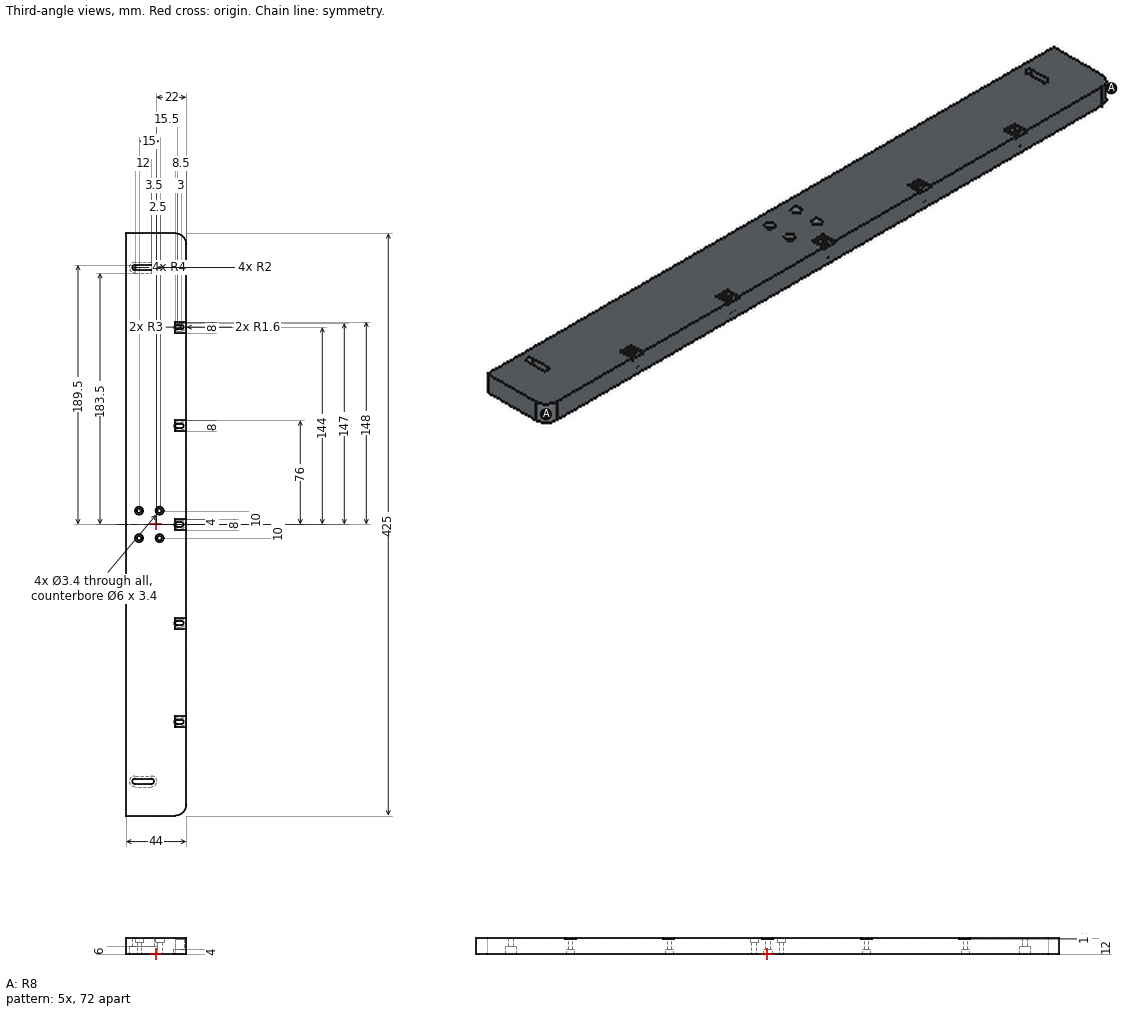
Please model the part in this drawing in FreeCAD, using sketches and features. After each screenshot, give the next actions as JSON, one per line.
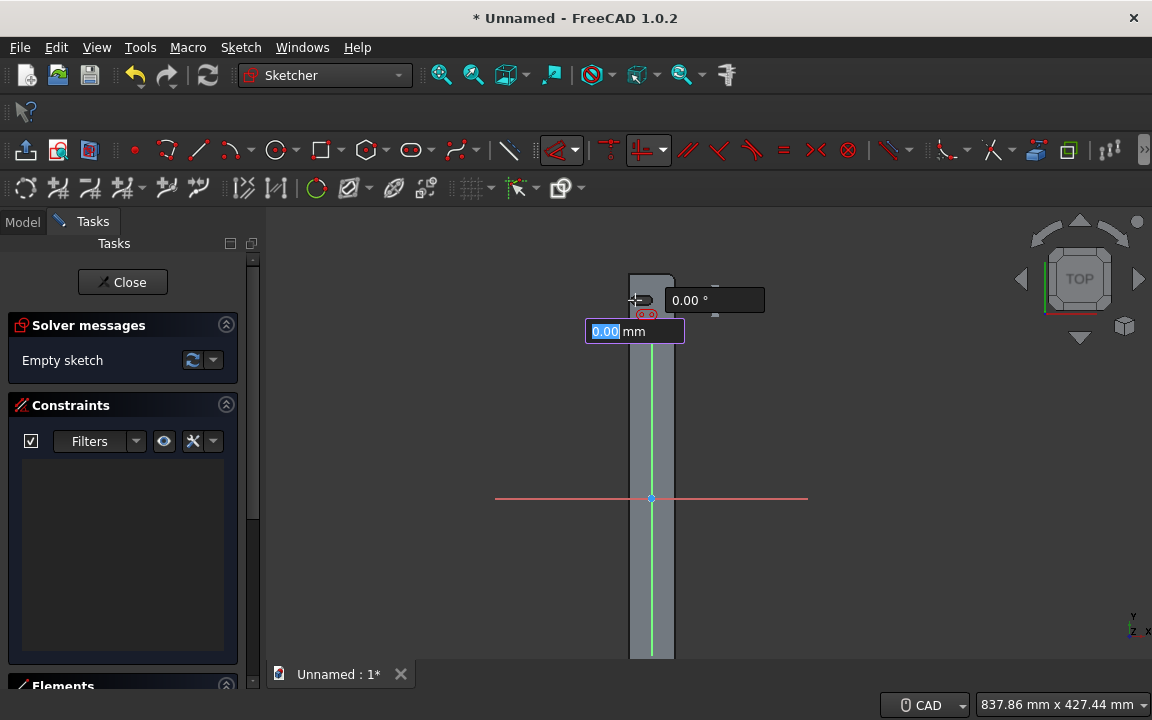
{"action": "scroll", "coordinate": [648, 300], "scroll_direction": "up", "scroll_amount": 8}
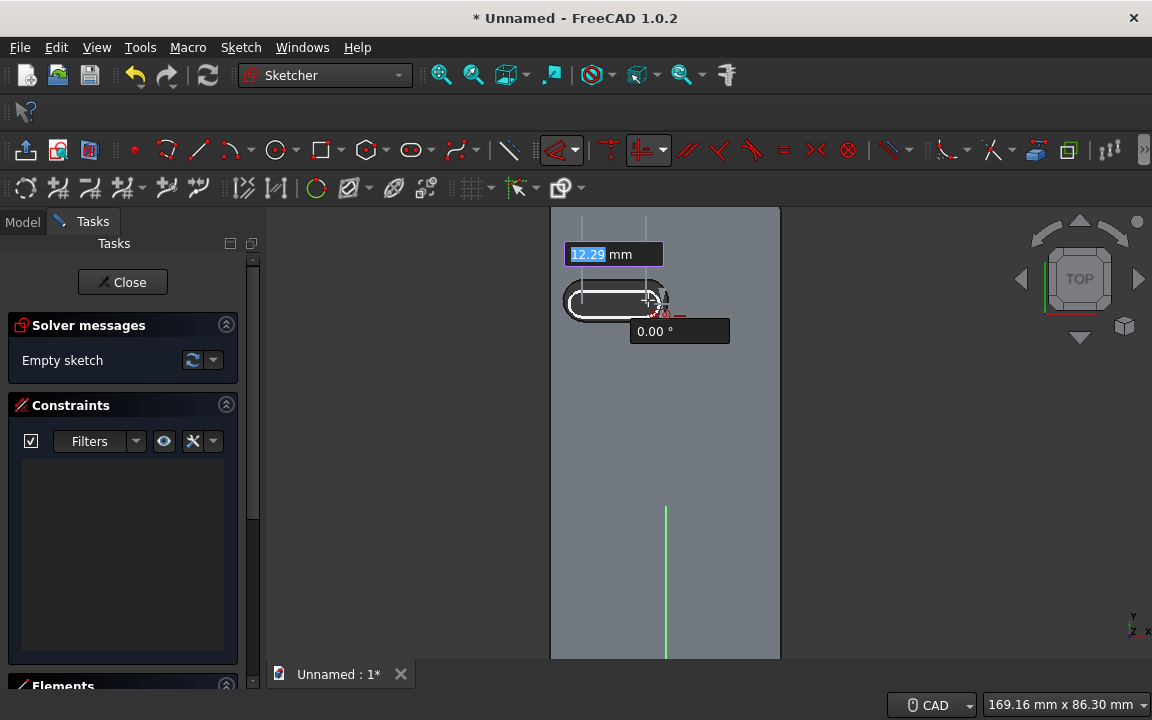
{"action": "left_click", "coordinate": [647, 299]}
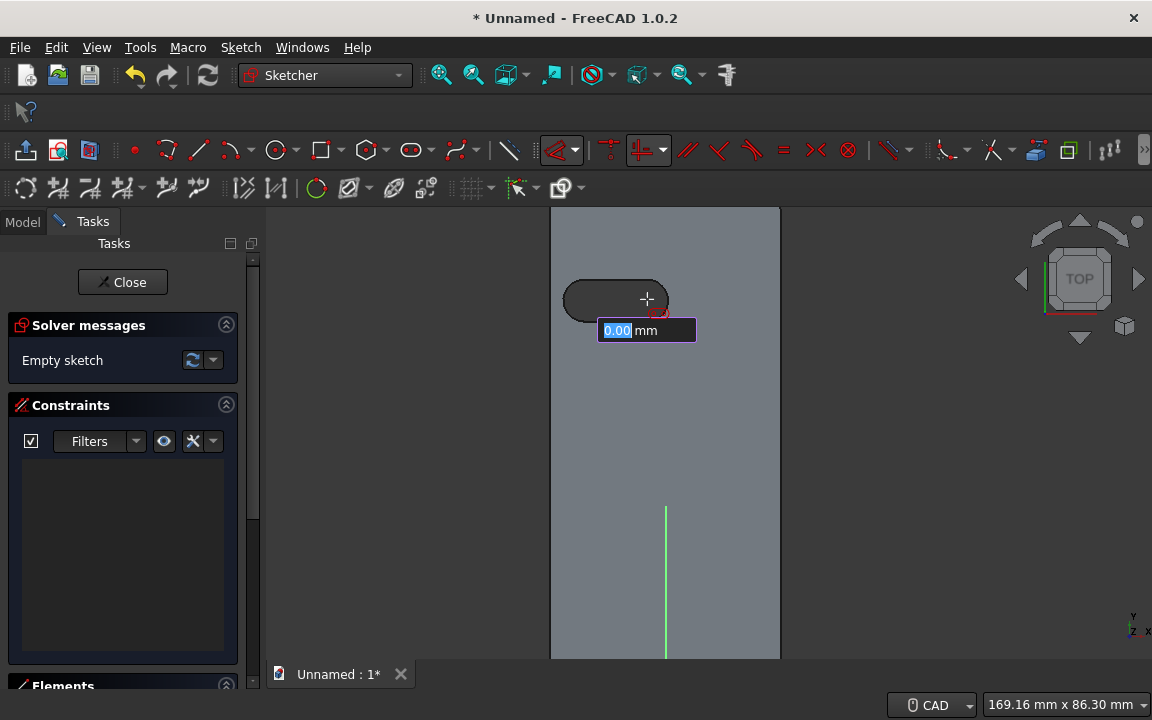
{"action": "scroll", "coordinate": [616, 290], "scroll_direction": "up", "scroll_amount": 3}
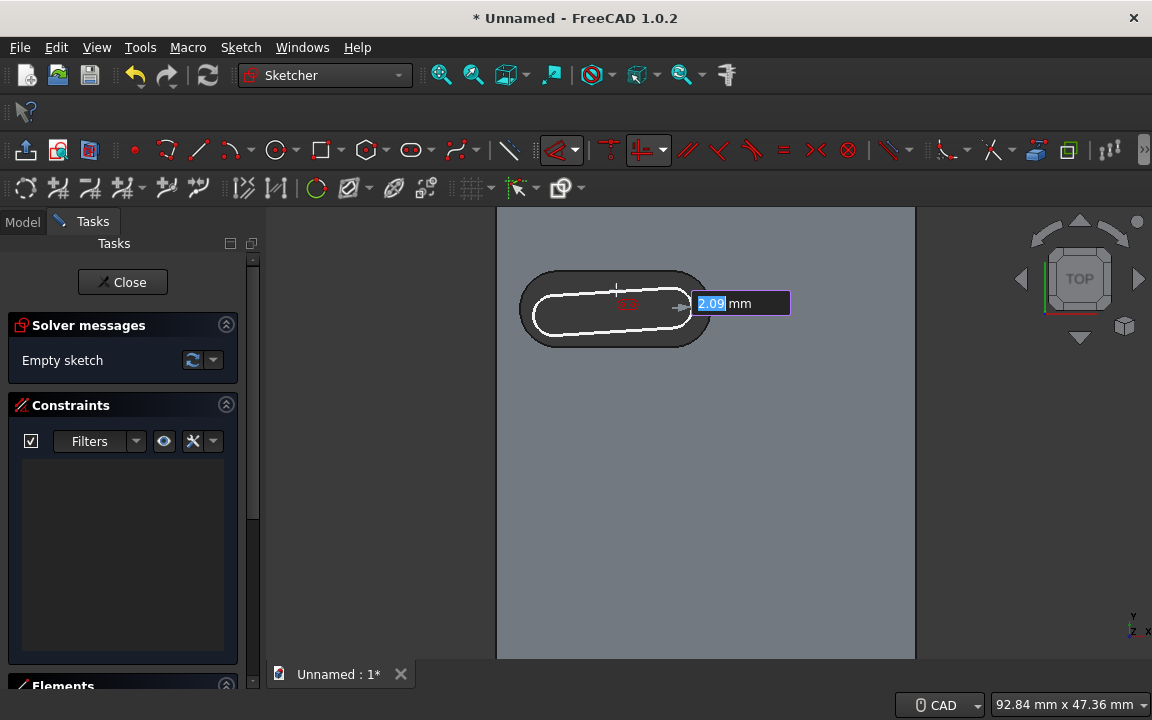
{"action": "left_click", "coordinate": [615, 290]}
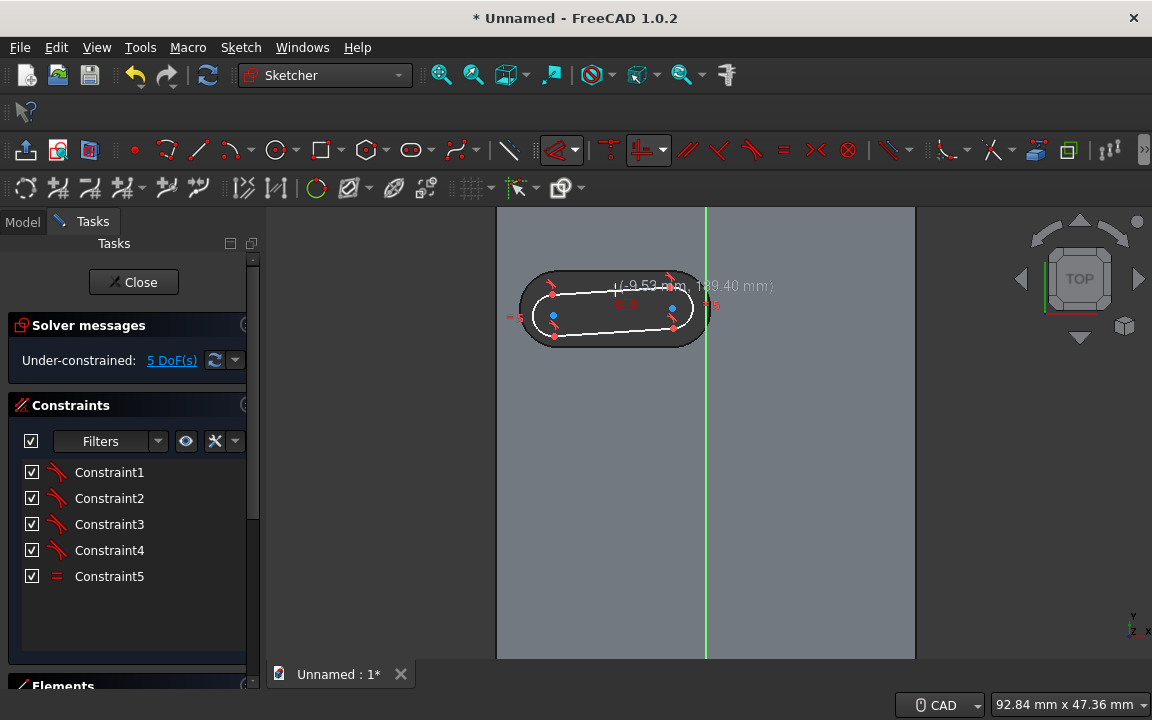
{"action": "scroll", "coordinate": [642, 299], "scroll_direction": "down", "scroll_amount": 13}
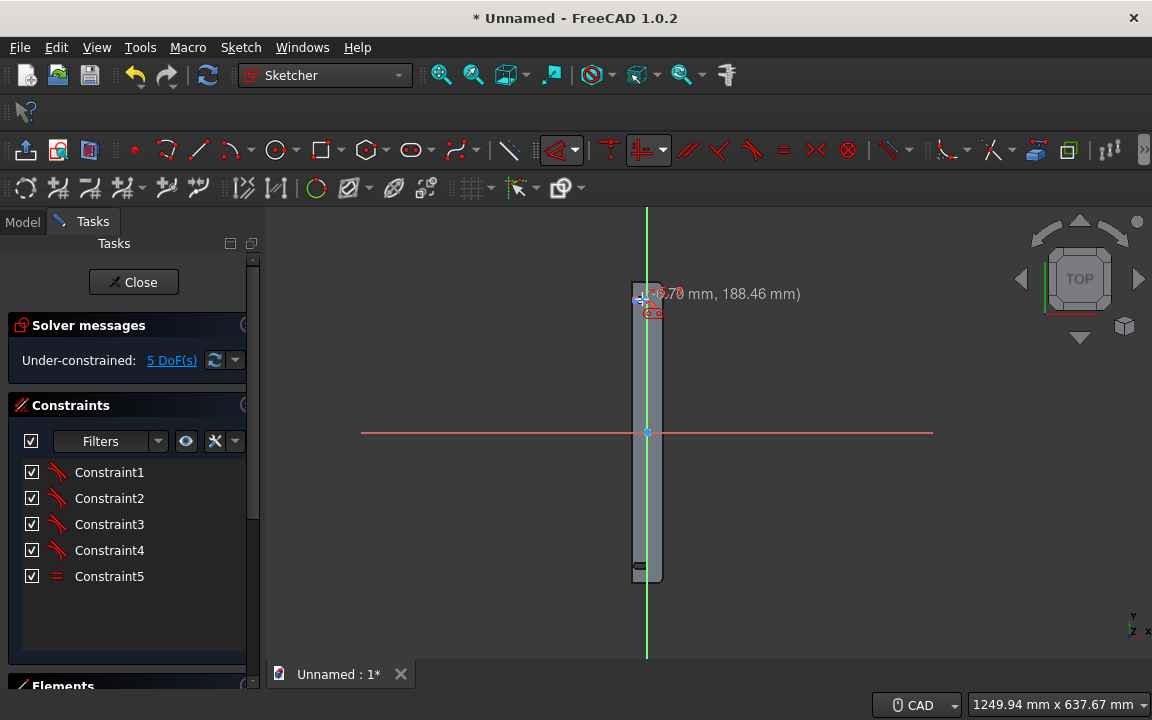
{"action": "scroll", "coordinate": [636, 566], "scroll_direction": "up", "scroll_amount": 14}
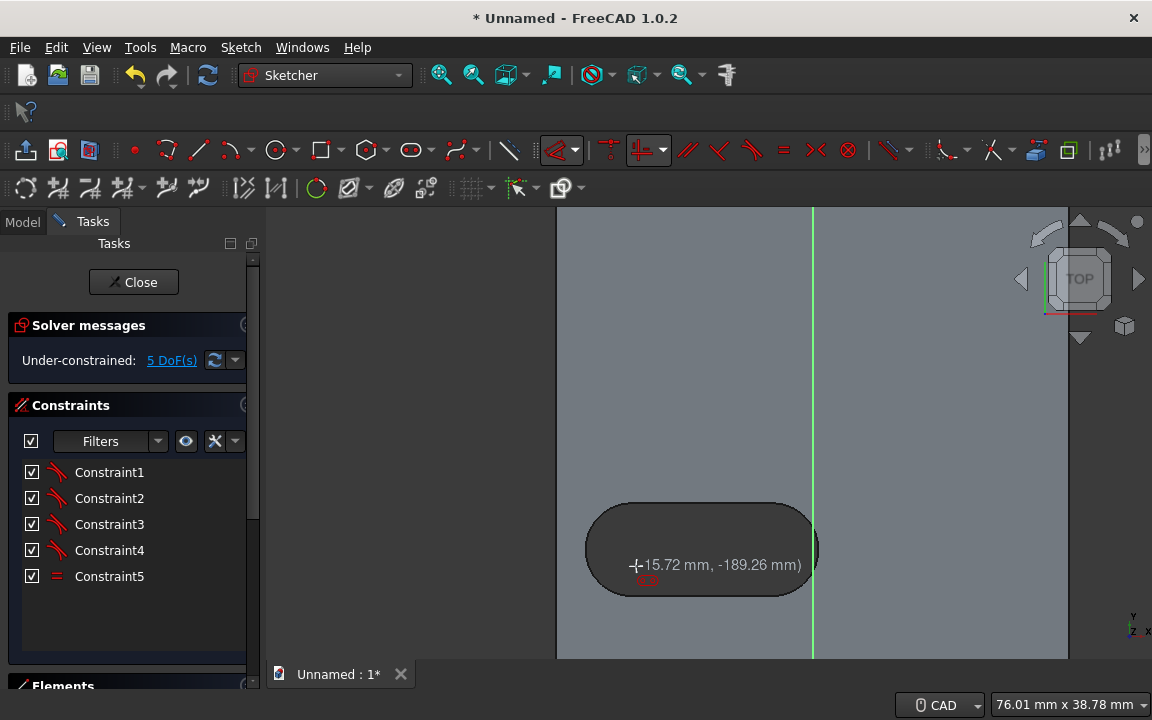
{"action": "scroll", "coordinate": [636, 567], "scroll_direction": "down", "scroll_amount": 14}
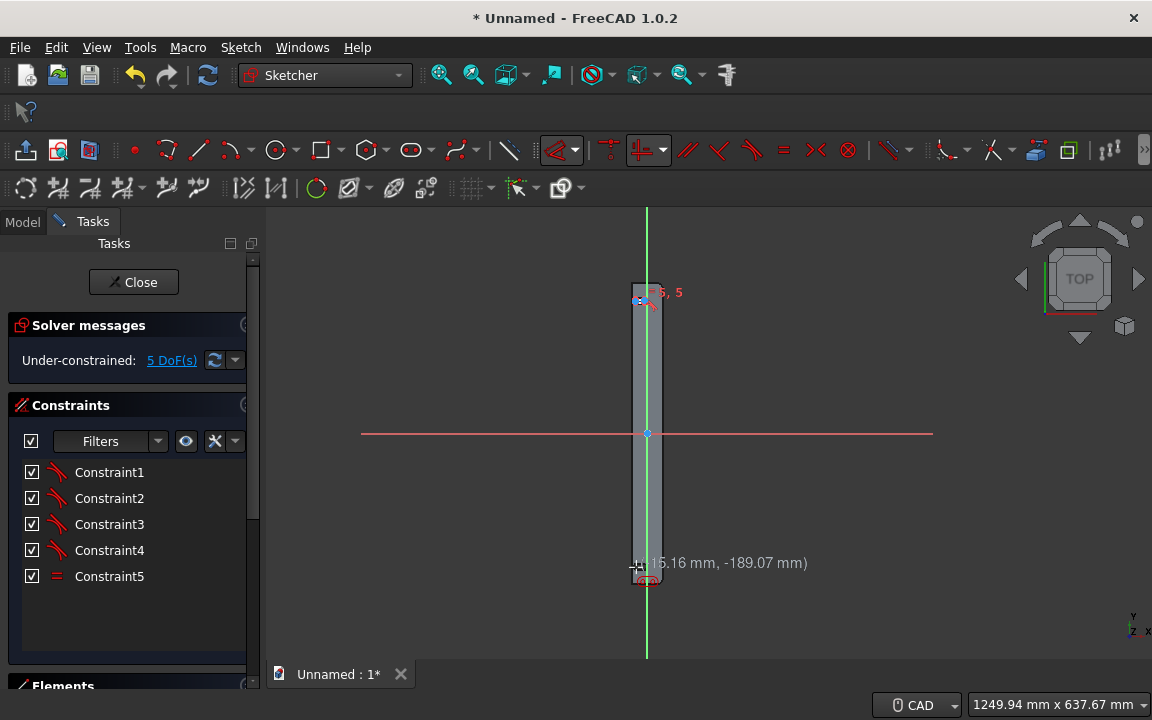
{"action": "scroll", "coordinate": [636, 567], "scroll_direction": "up", "scroll_amount": 2}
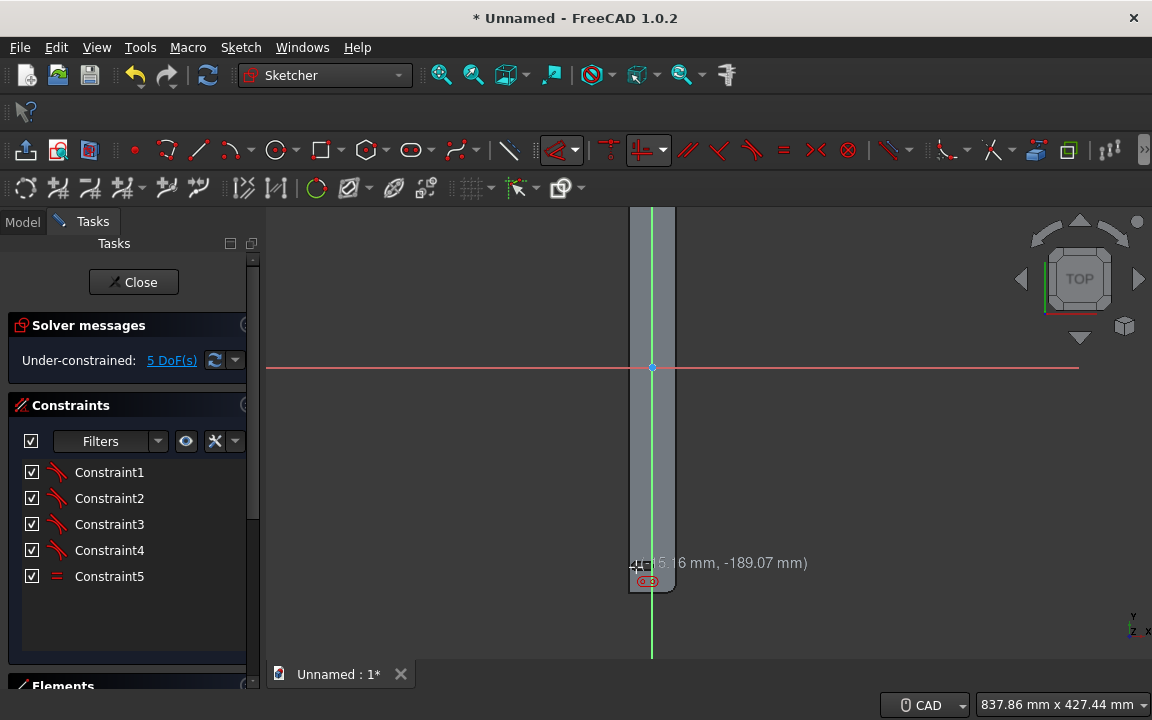
{"action": "left_click", "coordinate": [636, 566]}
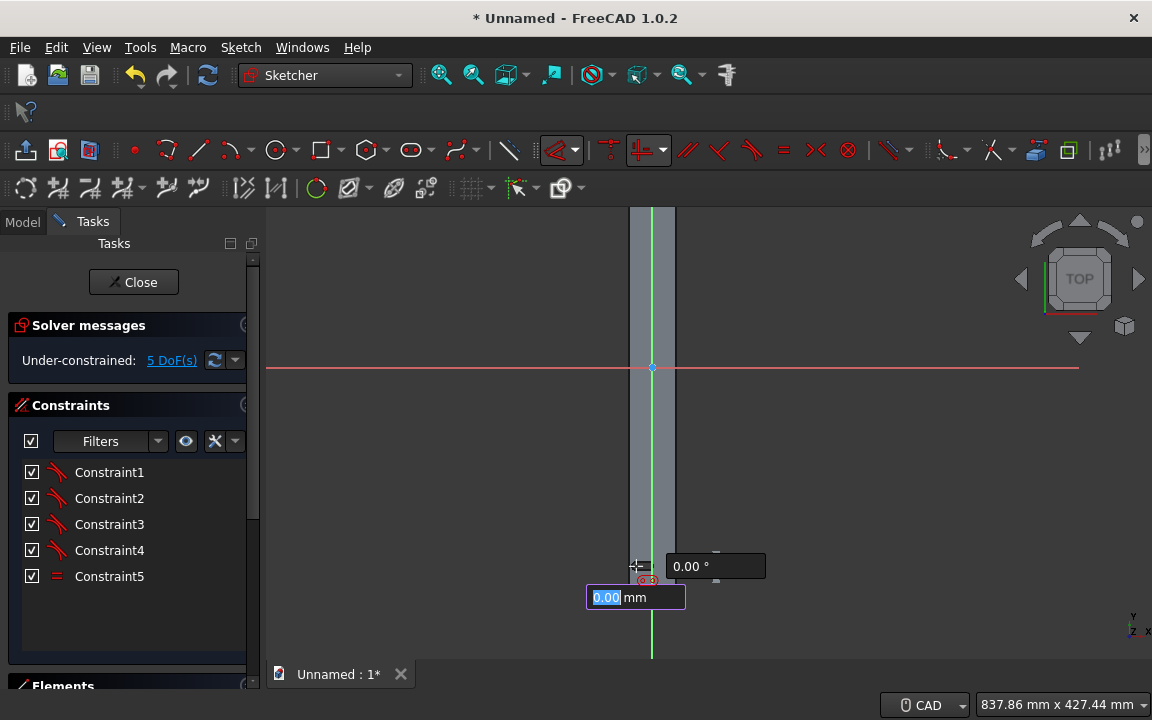
{"action": "scroll", "coordinate": [649, 566], "scroll_direction": "up", "scroll_amount": 8}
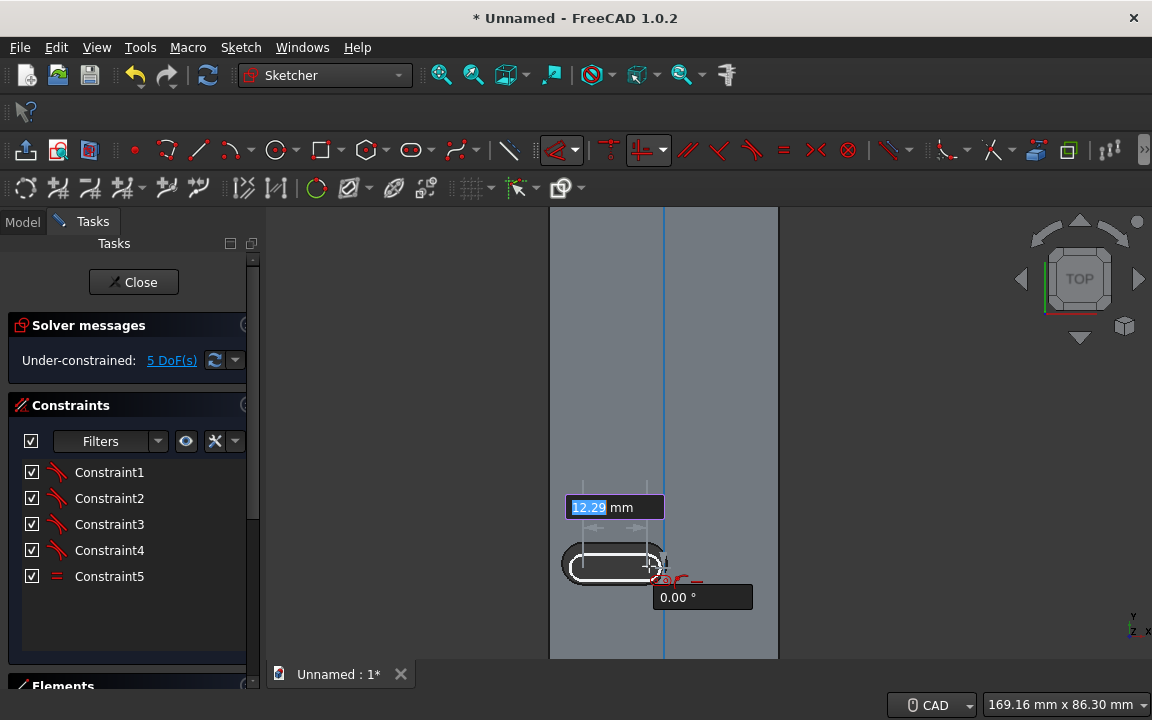
{"action": "left_click", "coordinate": [646, 563]}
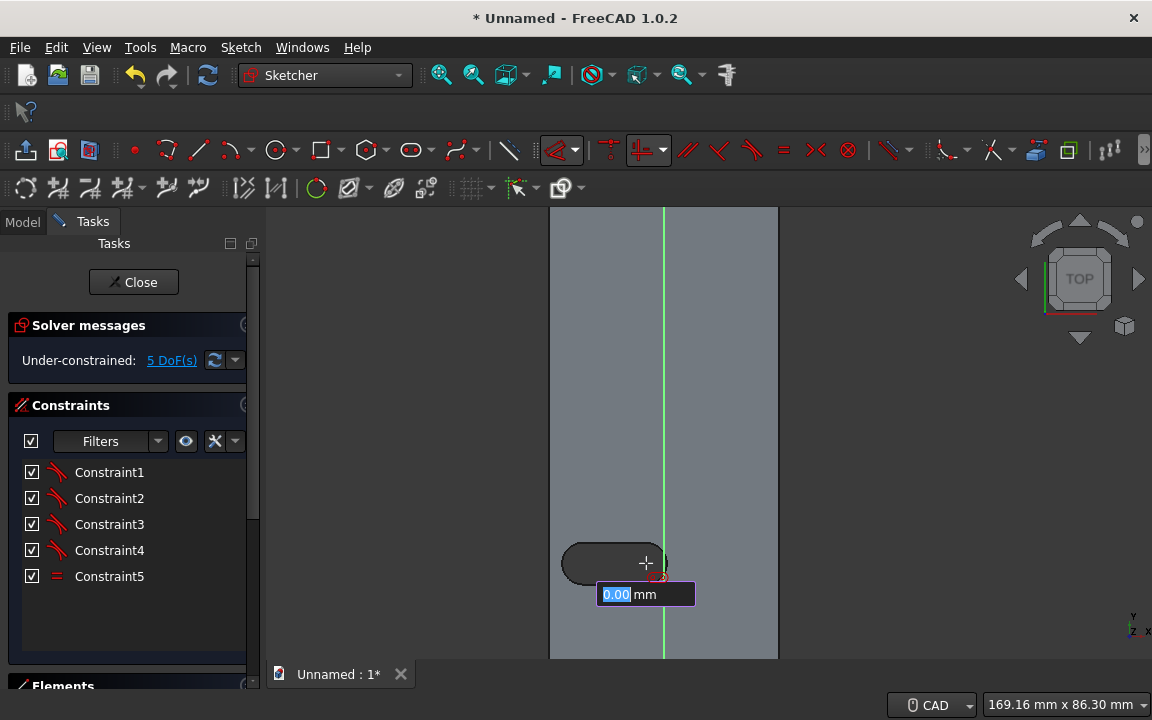
{"action": "scroll", "coordinate": [614, 574], "scroll_direction": "up", "scroll_amount": 3}